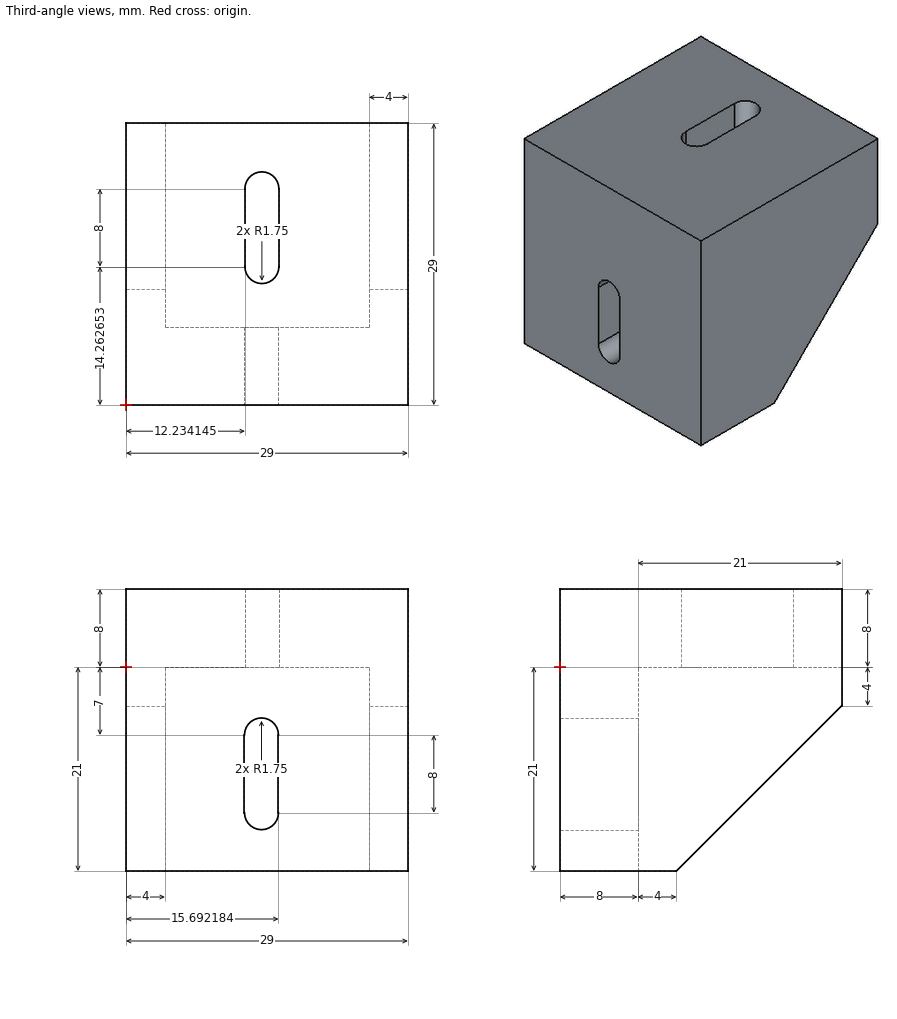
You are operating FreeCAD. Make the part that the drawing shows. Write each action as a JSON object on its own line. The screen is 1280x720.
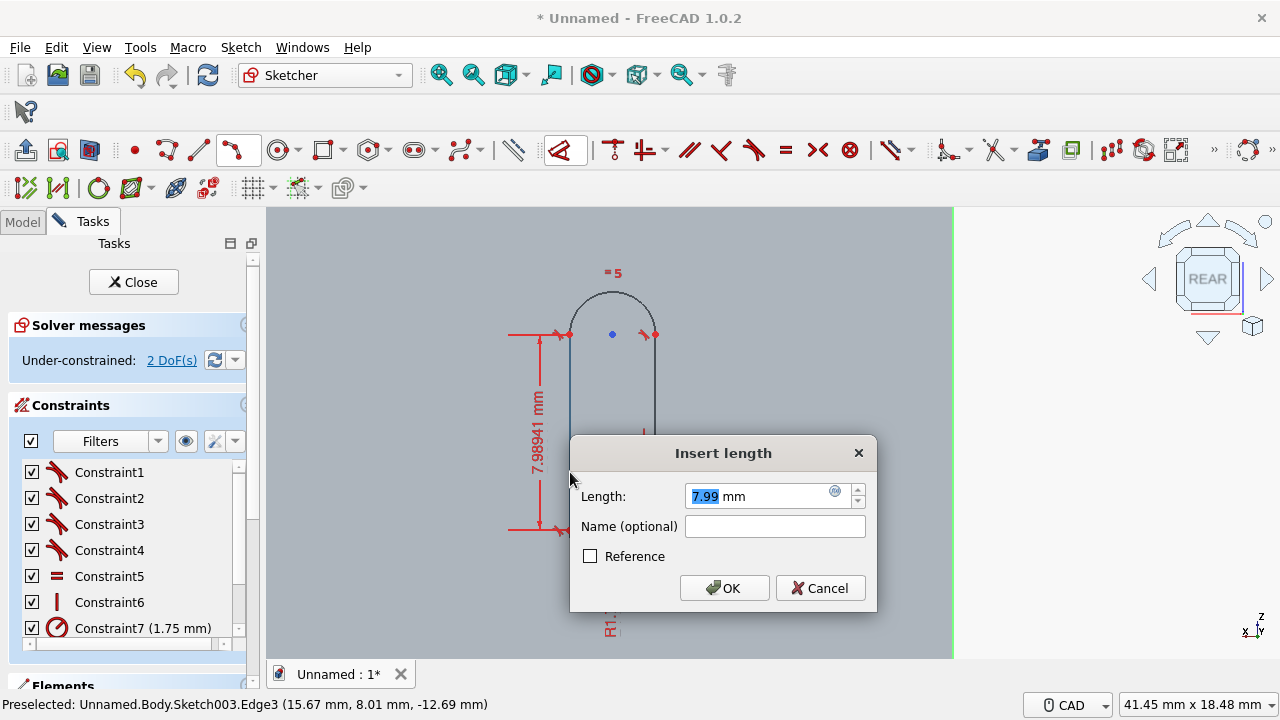
{"action": "type", "text": "8"}
{"action": "key", "text": "Return"}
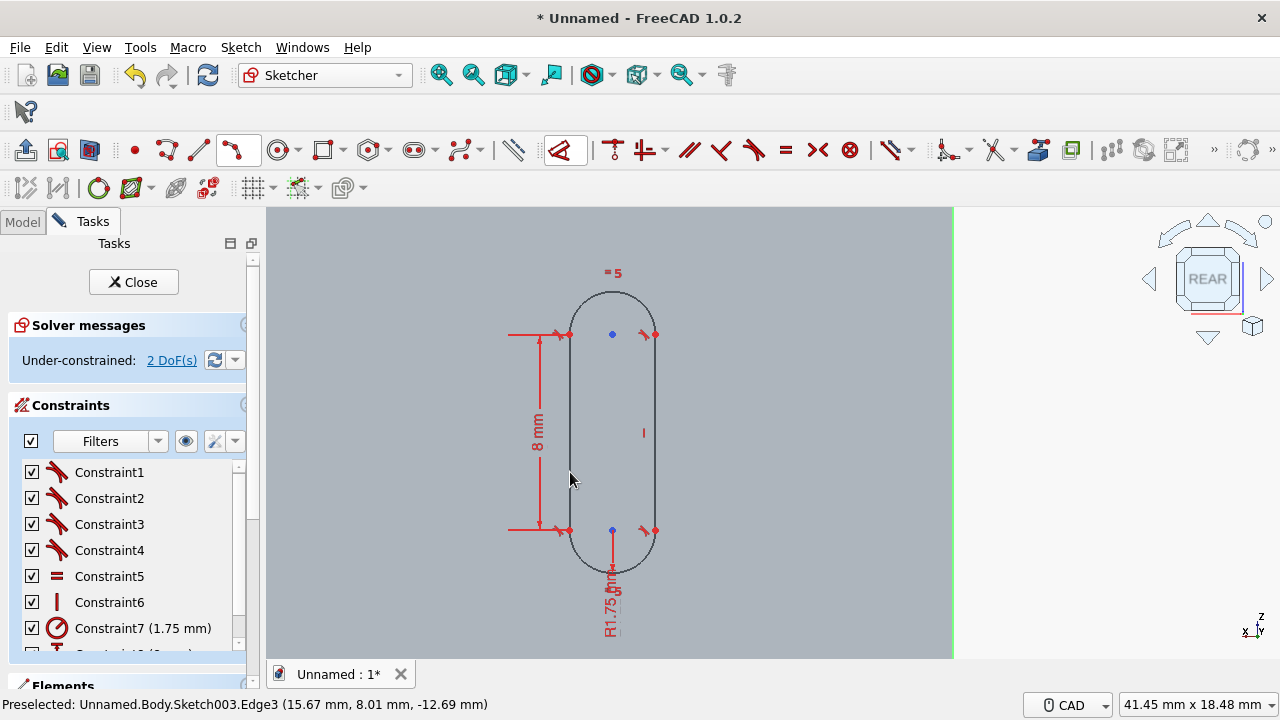
{"action": "left_click", "coordinate": [655, 335]}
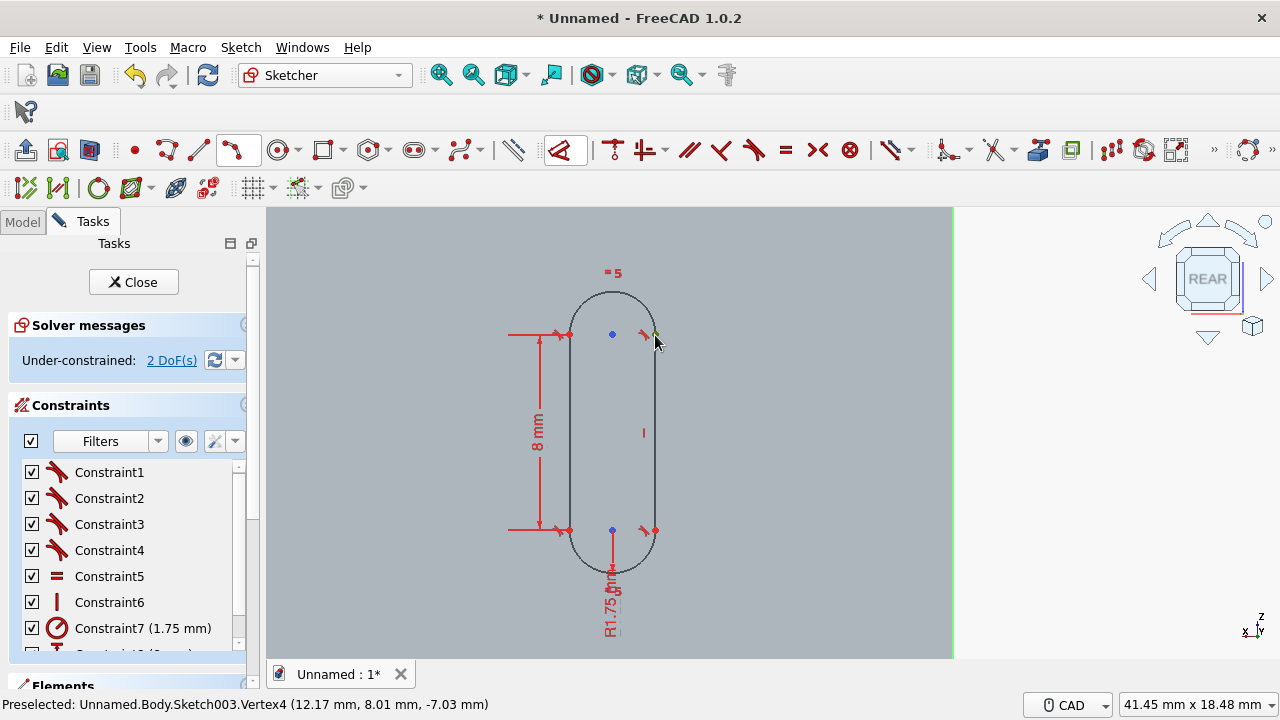
{"action": "key", "text": "i"}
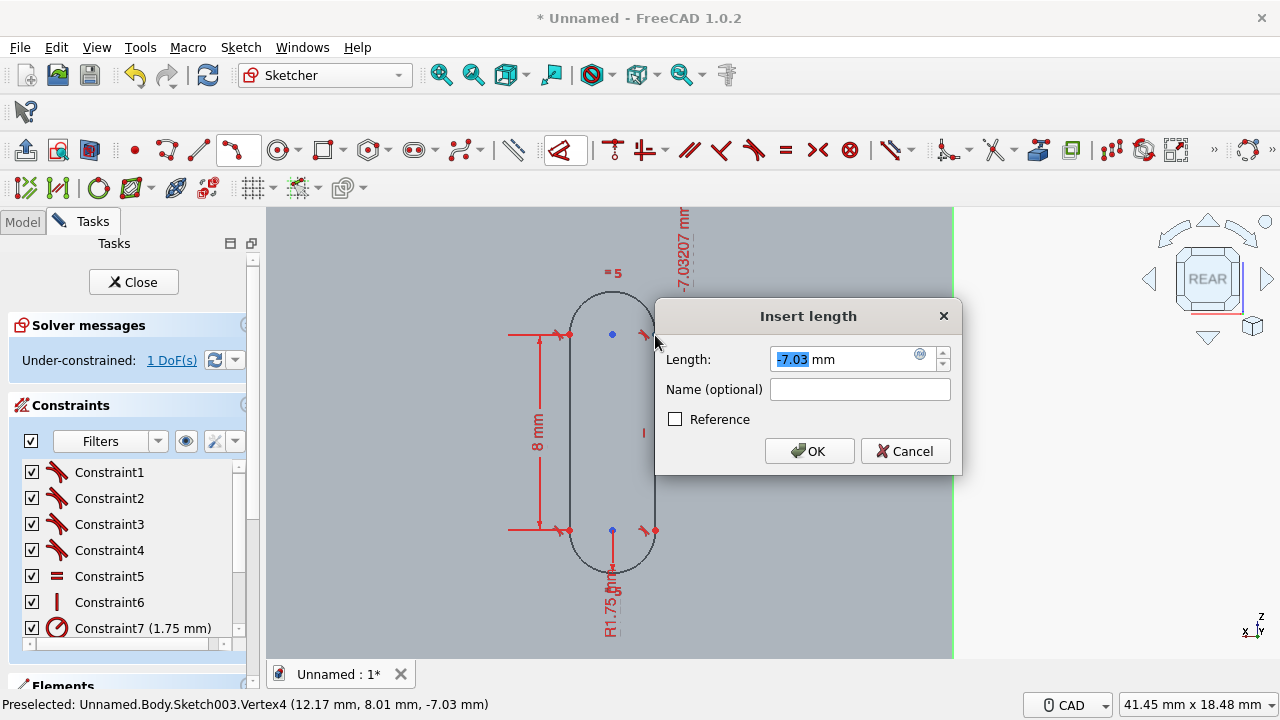
{"action": "type", "text": "-7"}
{"action": "key", "text": "Return"}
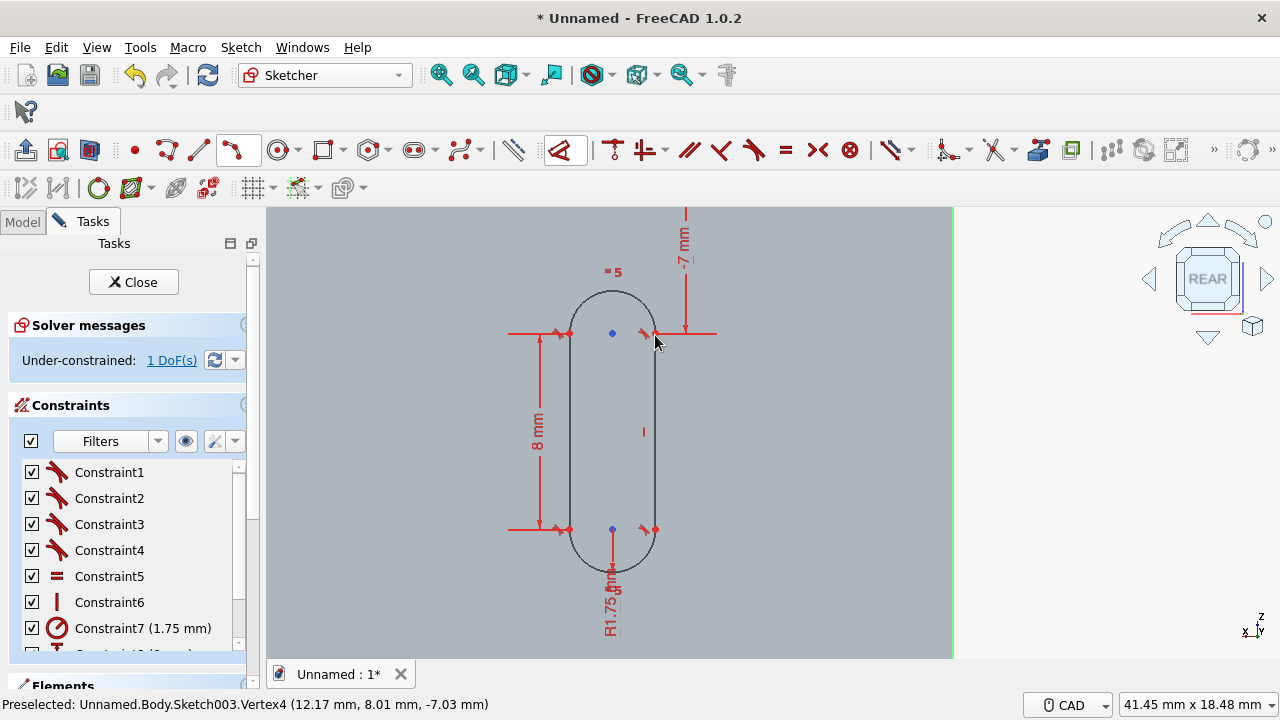
{"action": "left_click", "coordinate": [570, 530]}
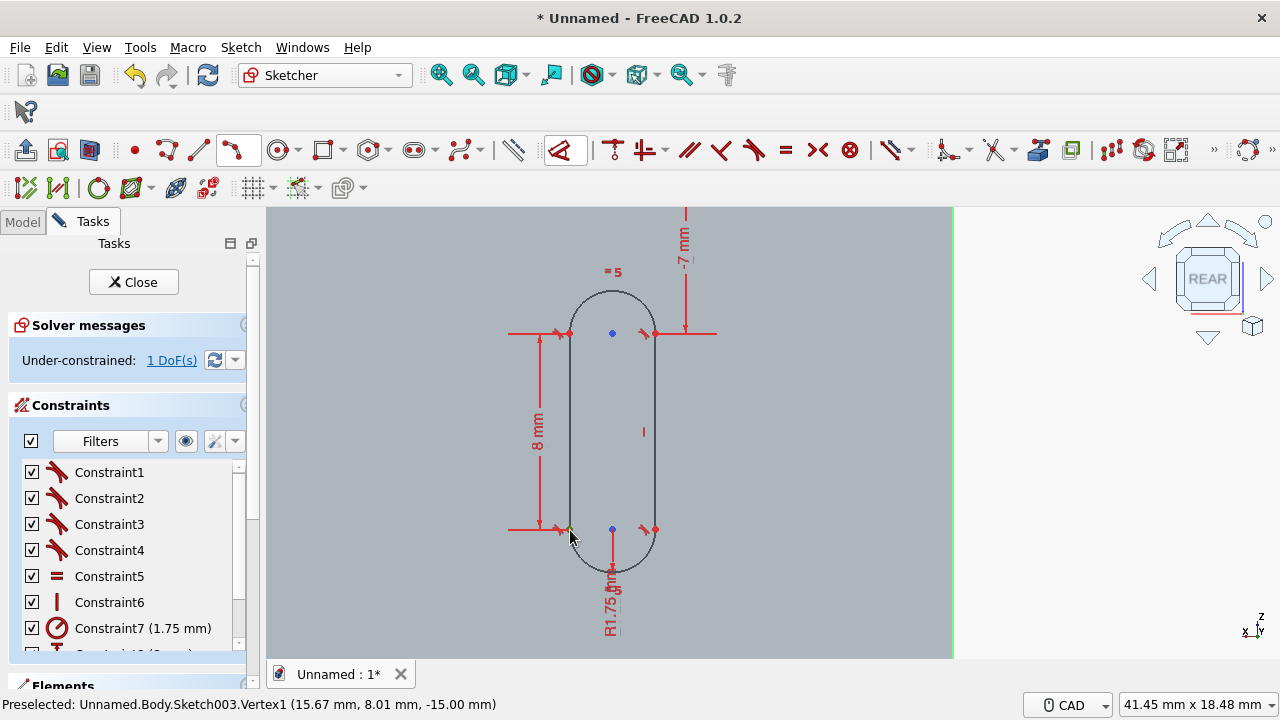
{"action": "left_click", "coordinate": [582, 150]}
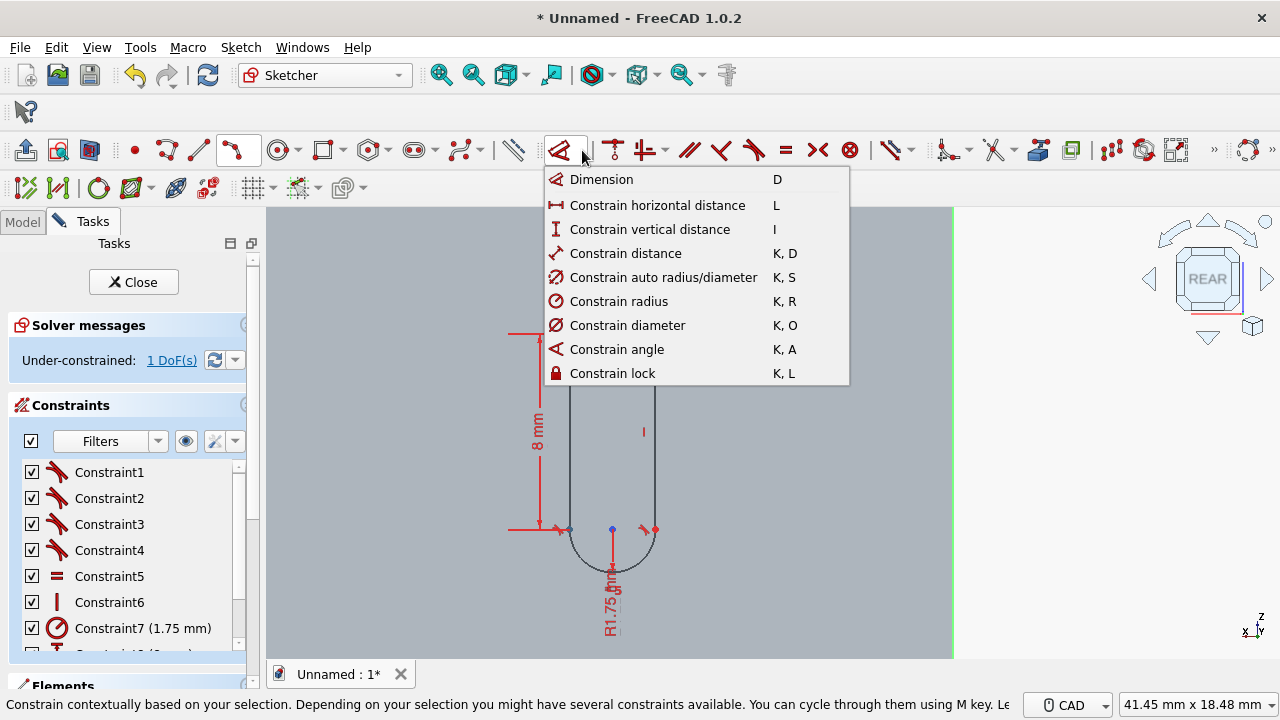
{"action": "left_click", "coordinate": [697, 205]}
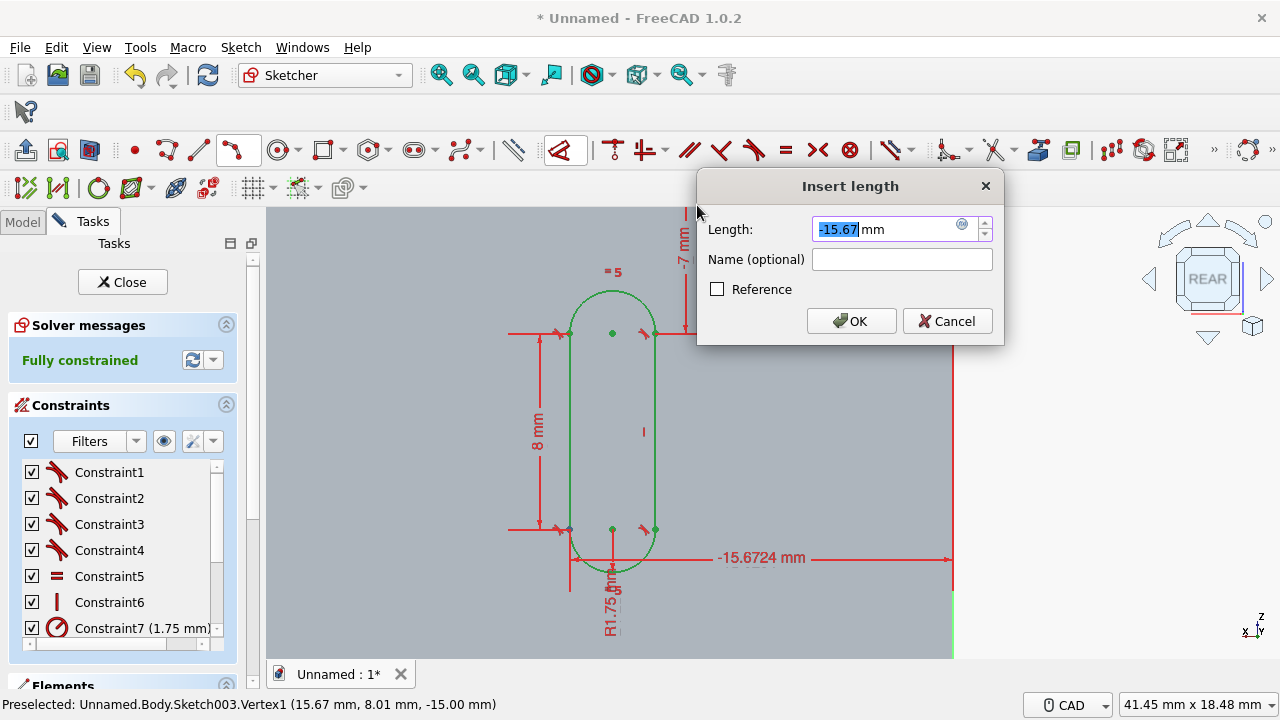
{"action": "type", "text": "-15.692184"}
{"action": "key", "text": "Return"}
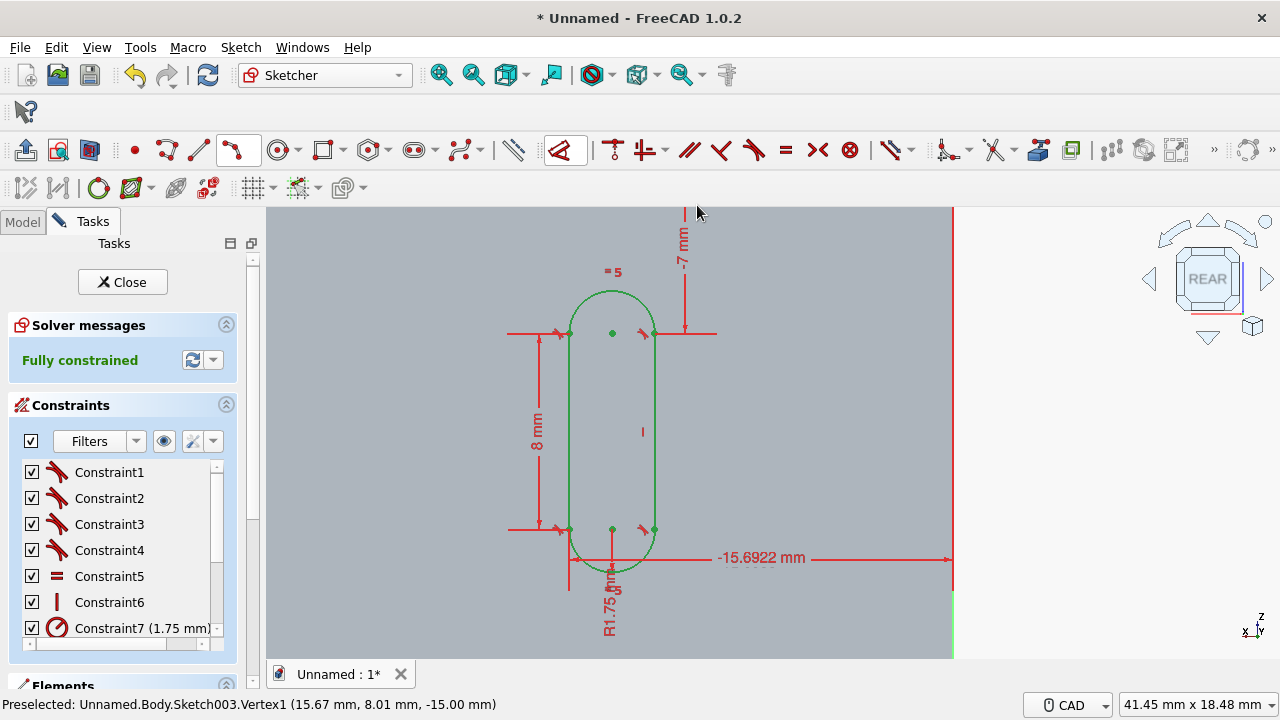
{"action": "left_click", "coordinate": [123, 282]}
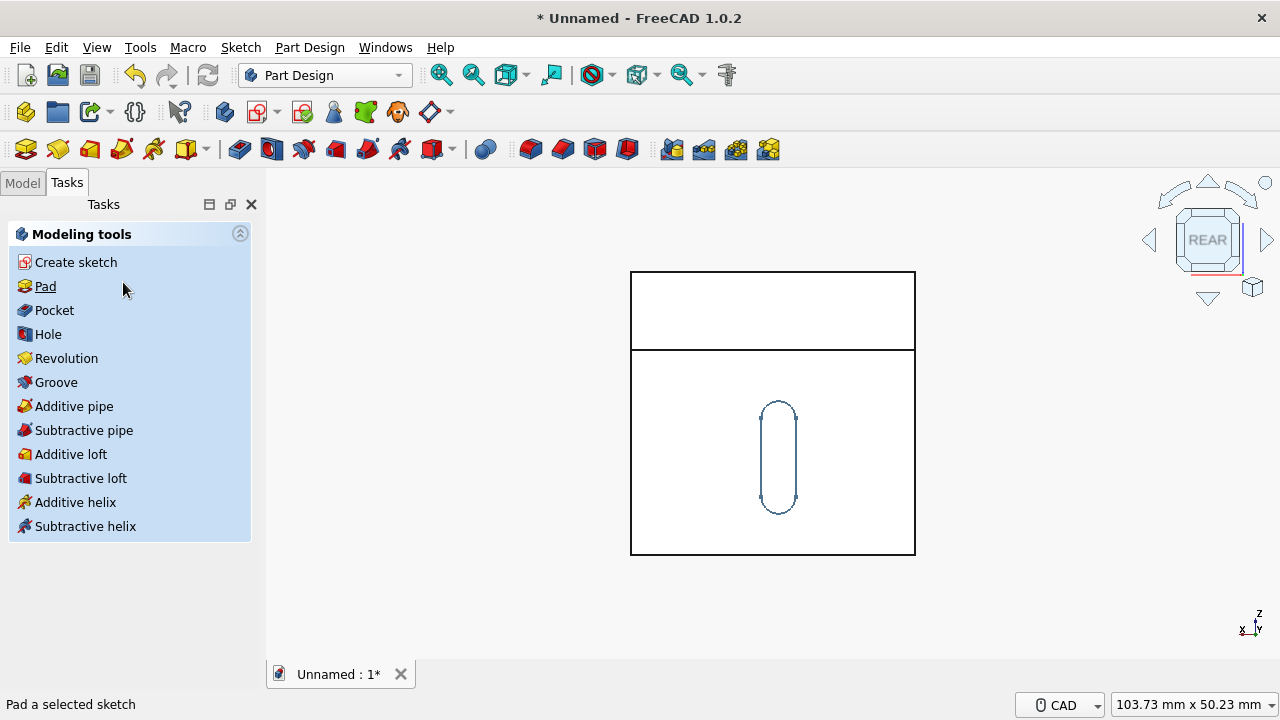
{"action": "left_click", "coordinate": [240, 150]}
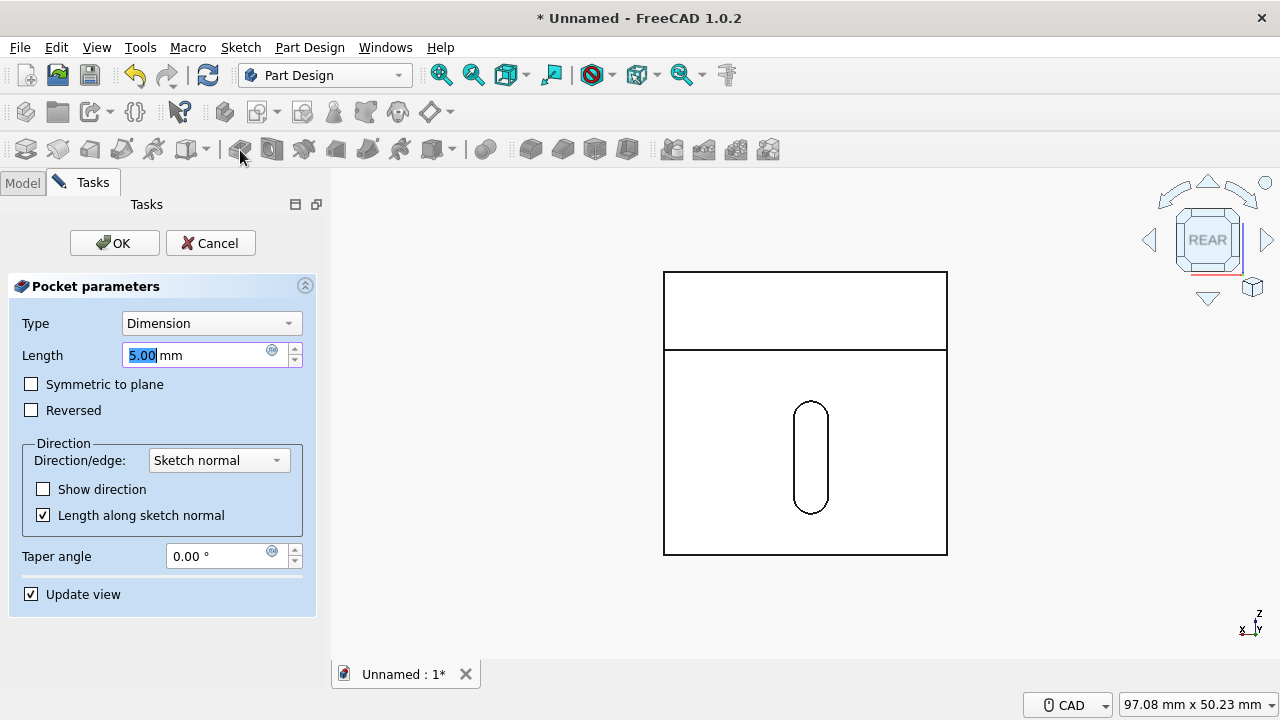
{"action": "type", "text": "8"}
{"action": "key", "text": "Tab"}